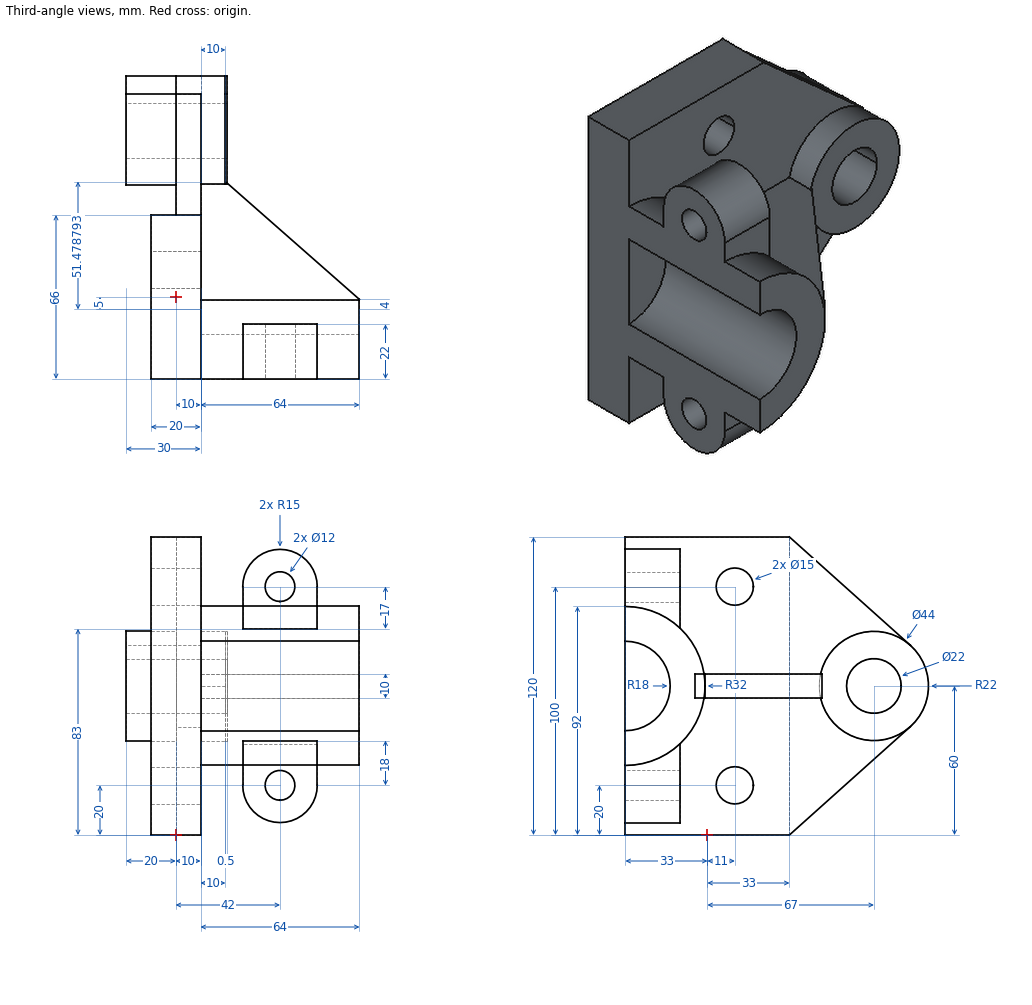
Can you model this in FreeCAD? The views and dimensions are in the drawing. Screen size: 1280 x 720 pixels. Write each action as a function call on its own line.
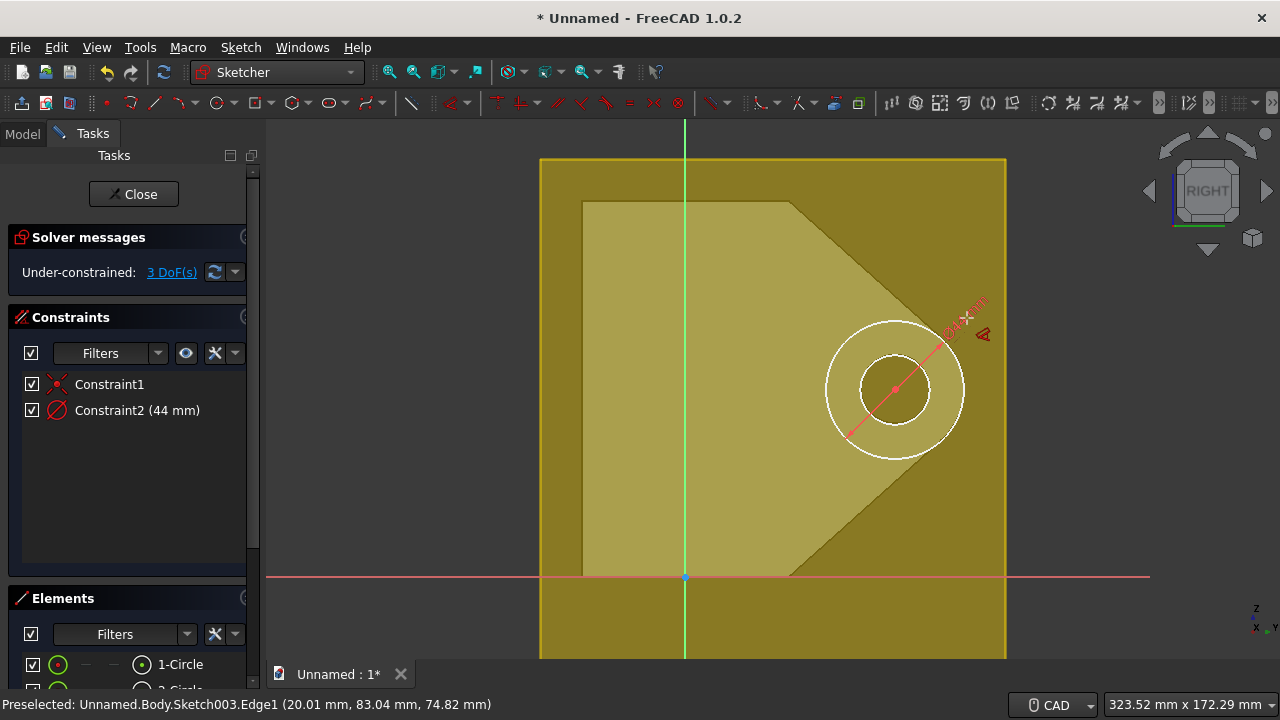
click(919, 365)
click(980, 363)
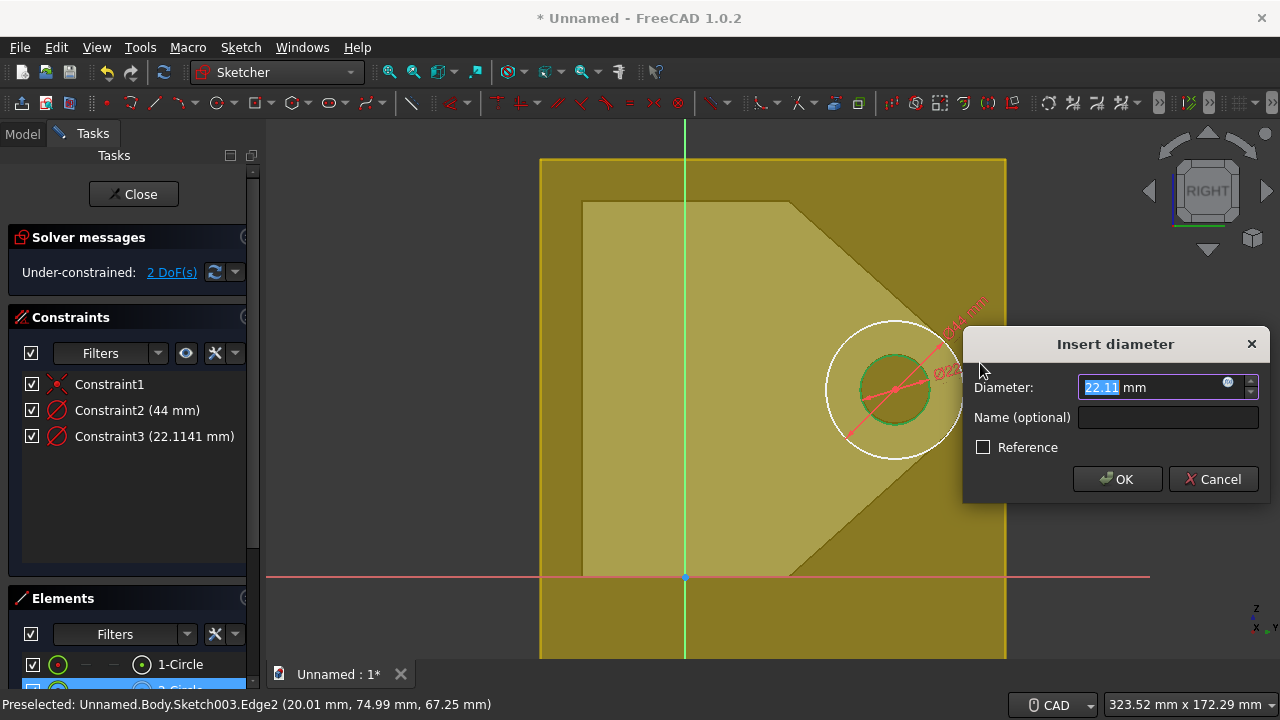
text(22)
key(Return)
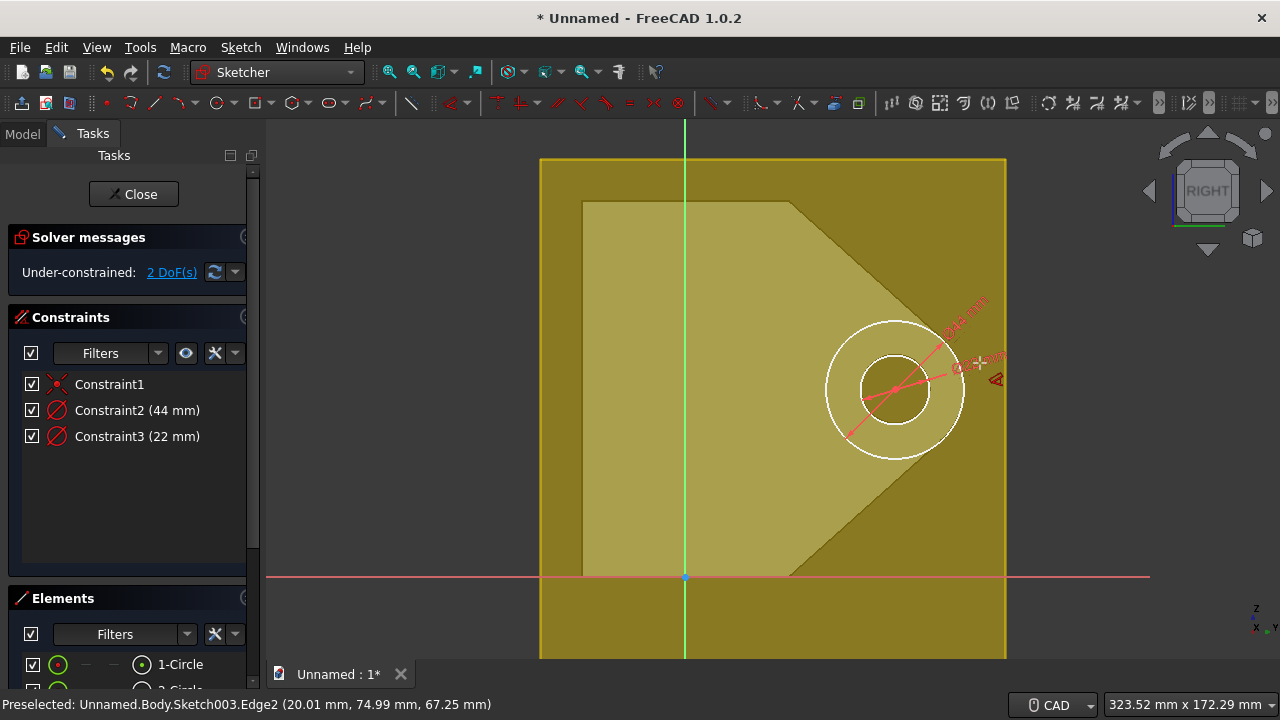
click(895, 390)
click(790, 611)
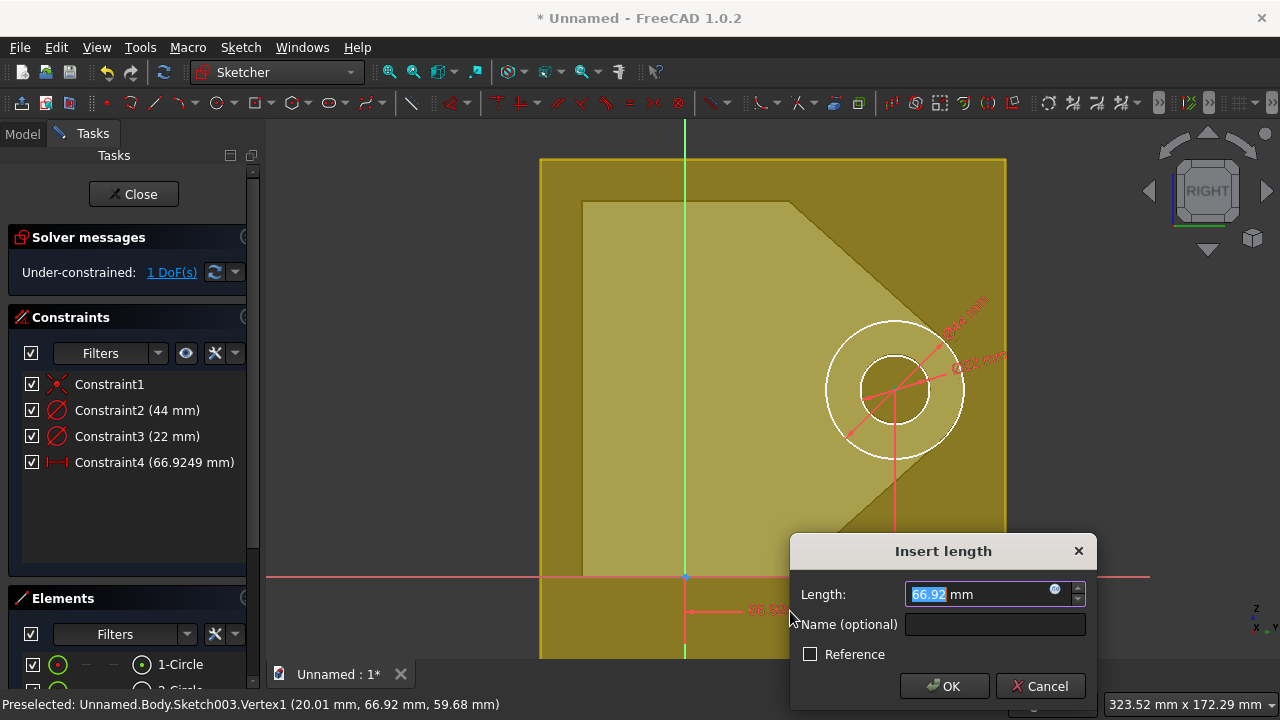
text(67)
key(Return)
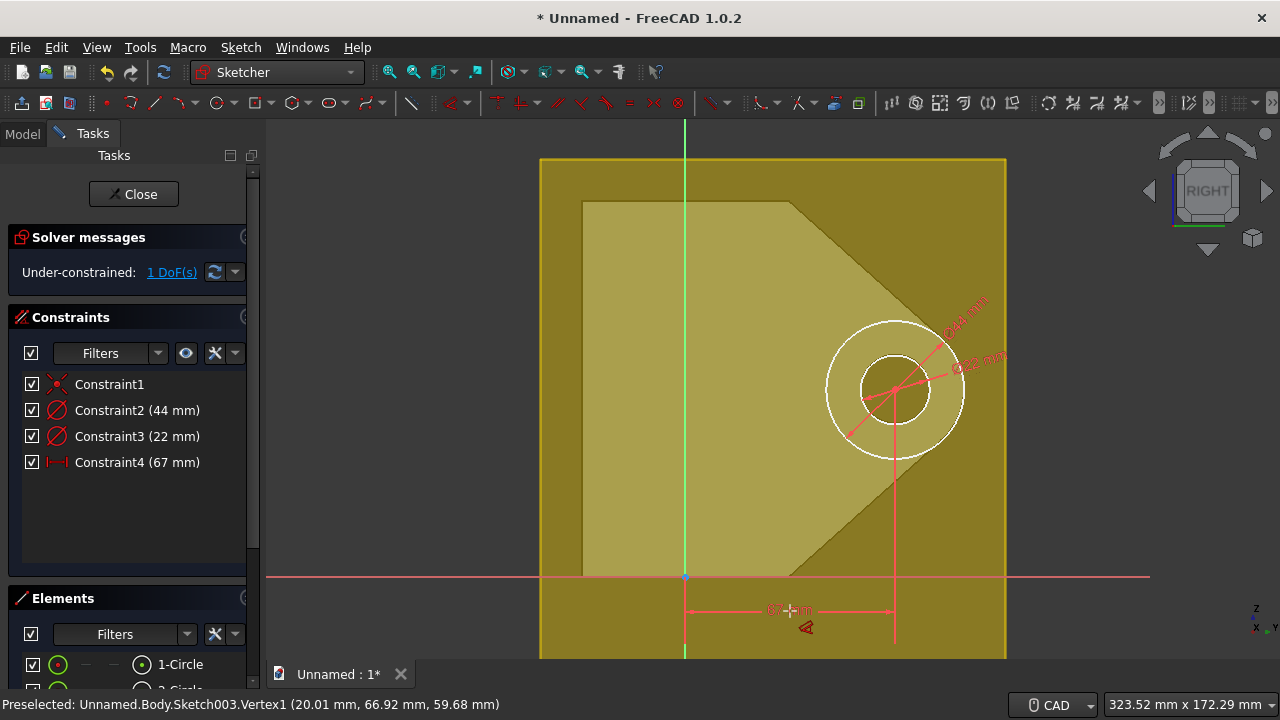
click(895, 390)
click(651, 484)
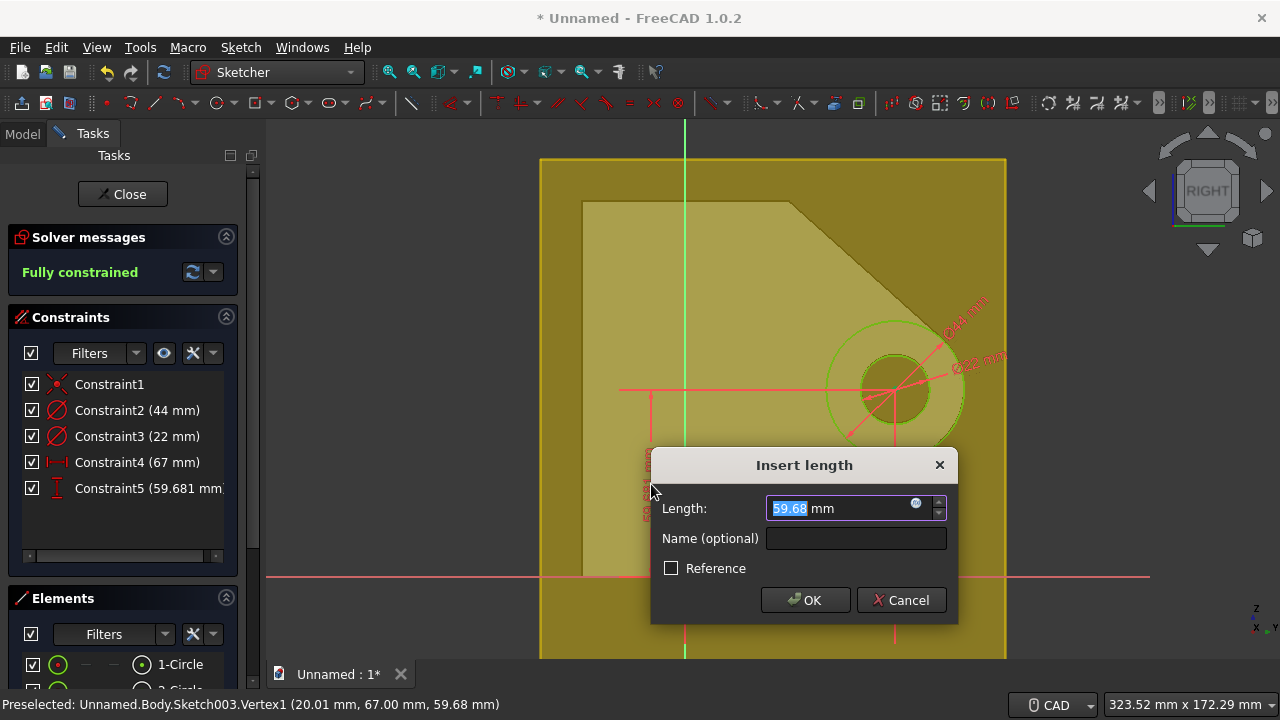
text(60)
key(Return)
key(Escape)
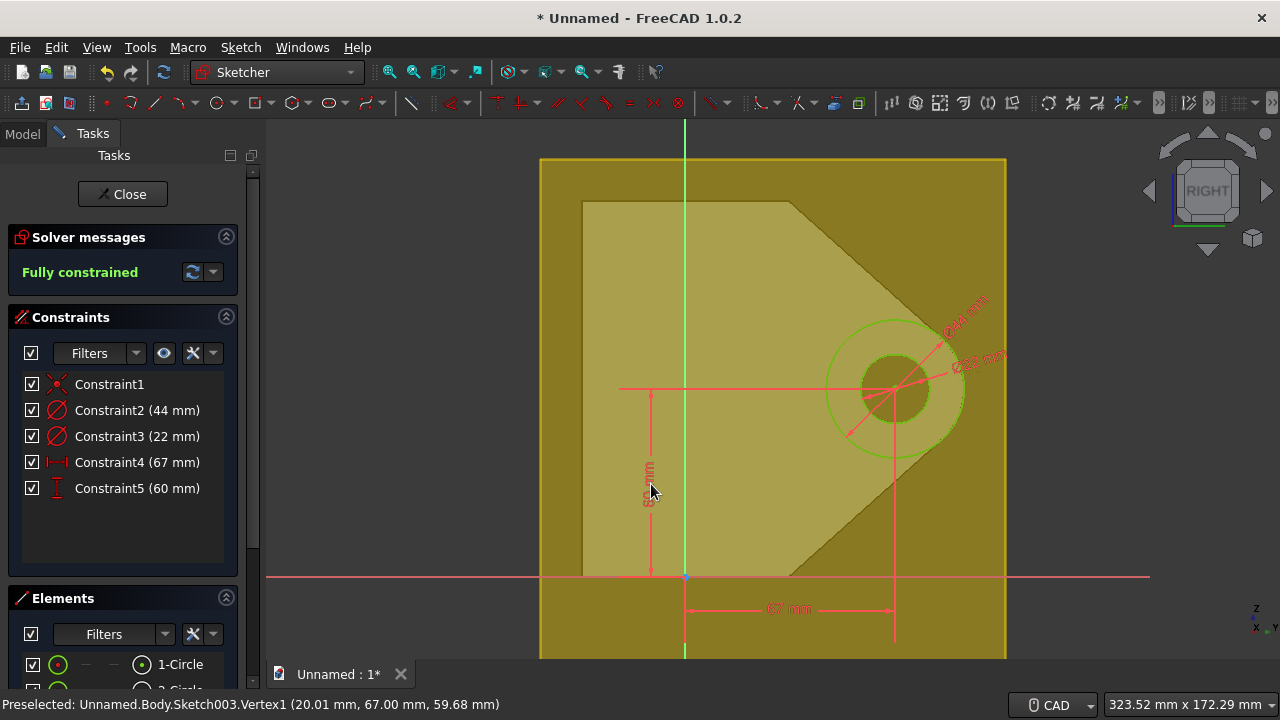
click(123, 194)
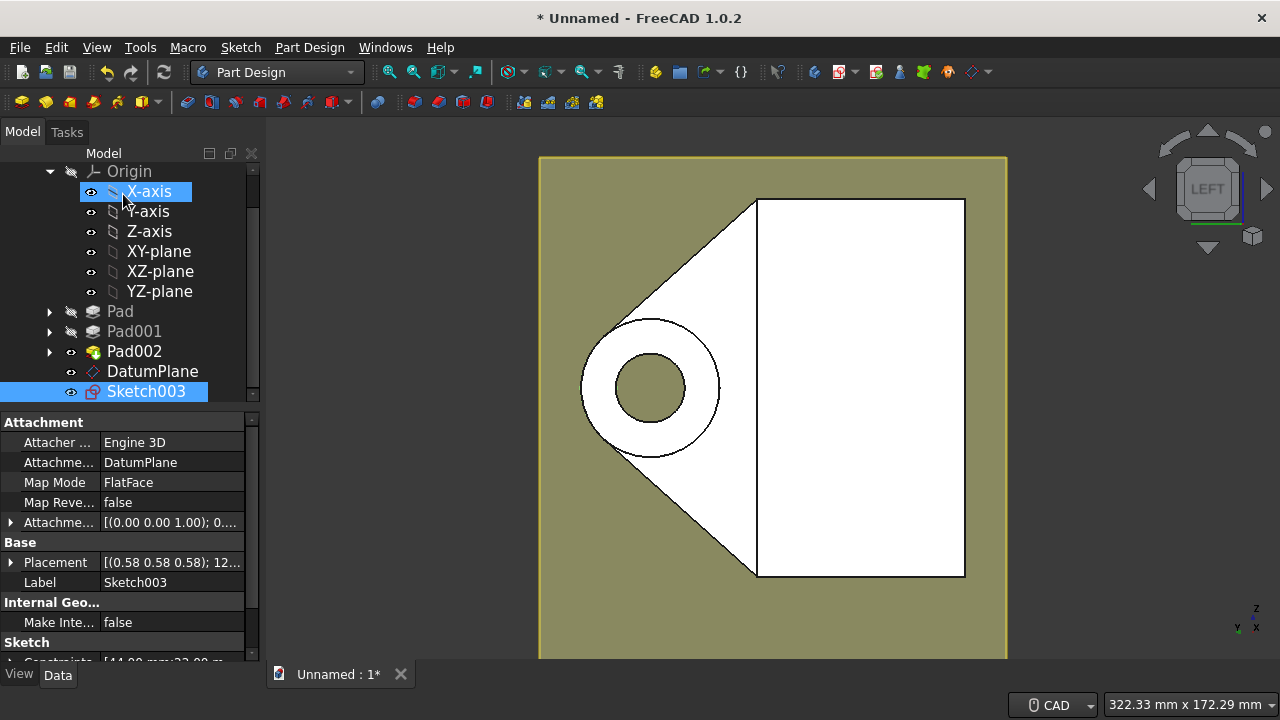
click(22, 102)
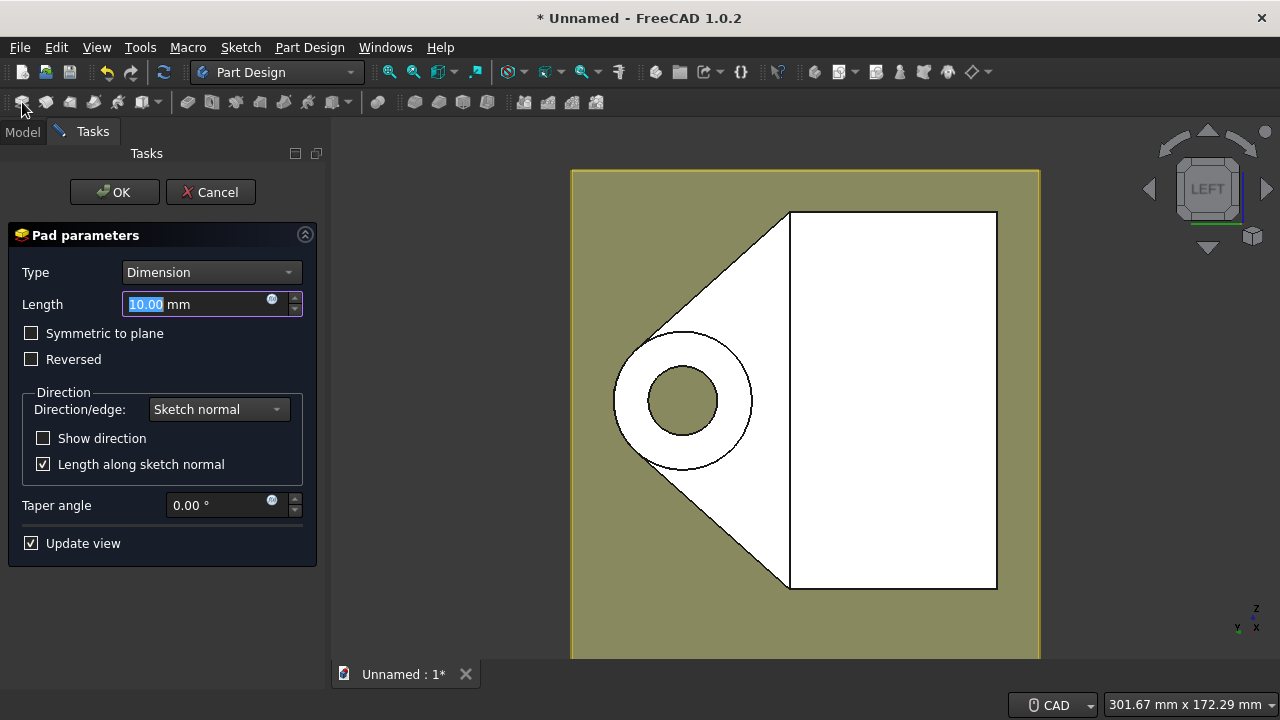
text(10)
key(Tab)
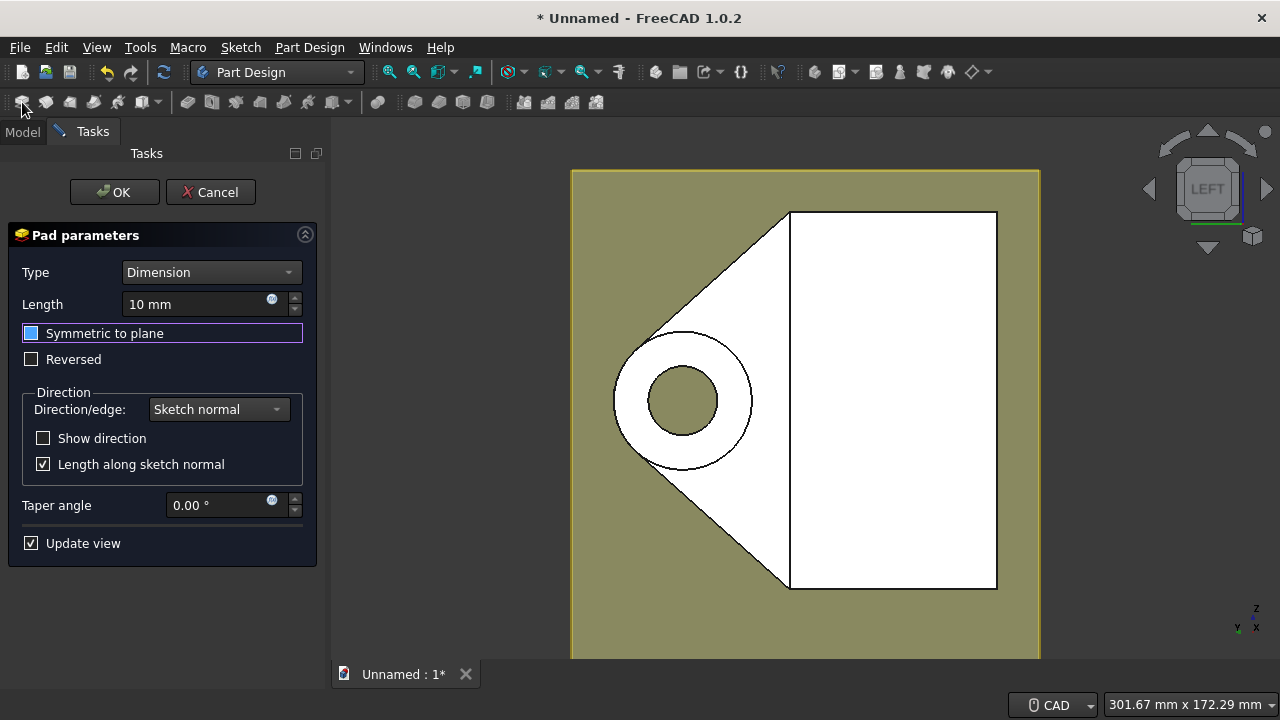
click(30, 359)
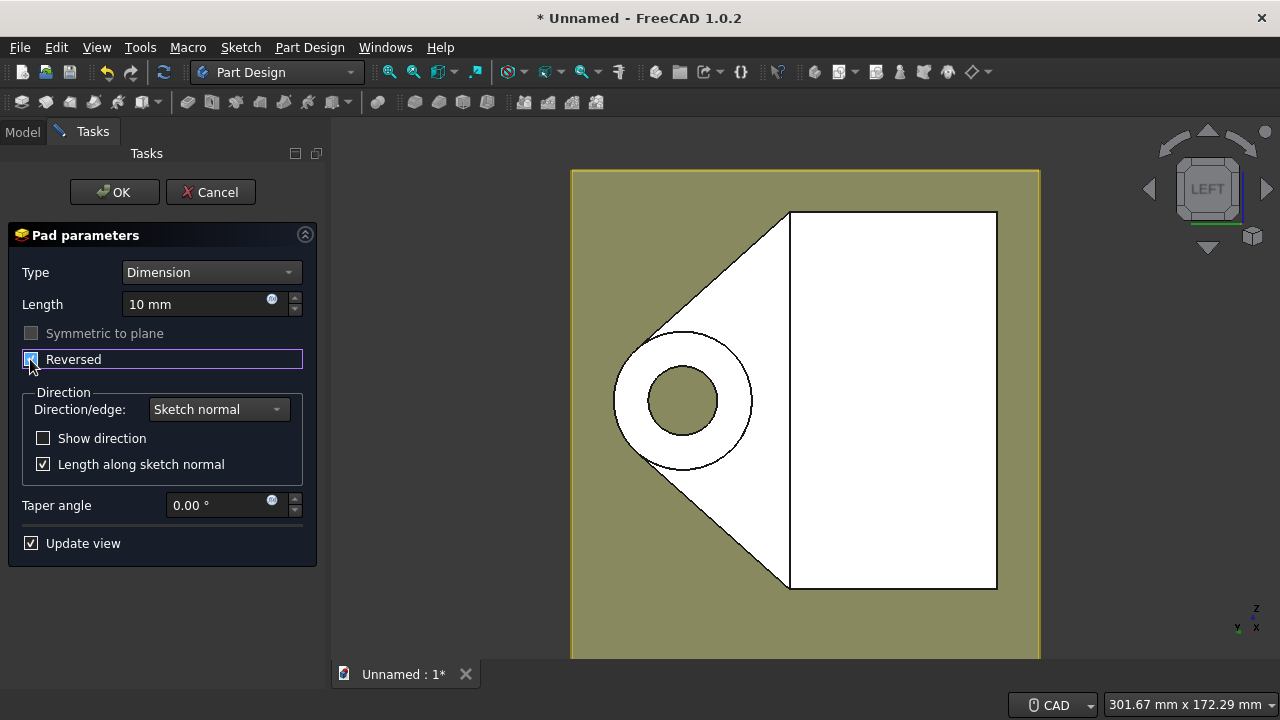
click(115, 192)